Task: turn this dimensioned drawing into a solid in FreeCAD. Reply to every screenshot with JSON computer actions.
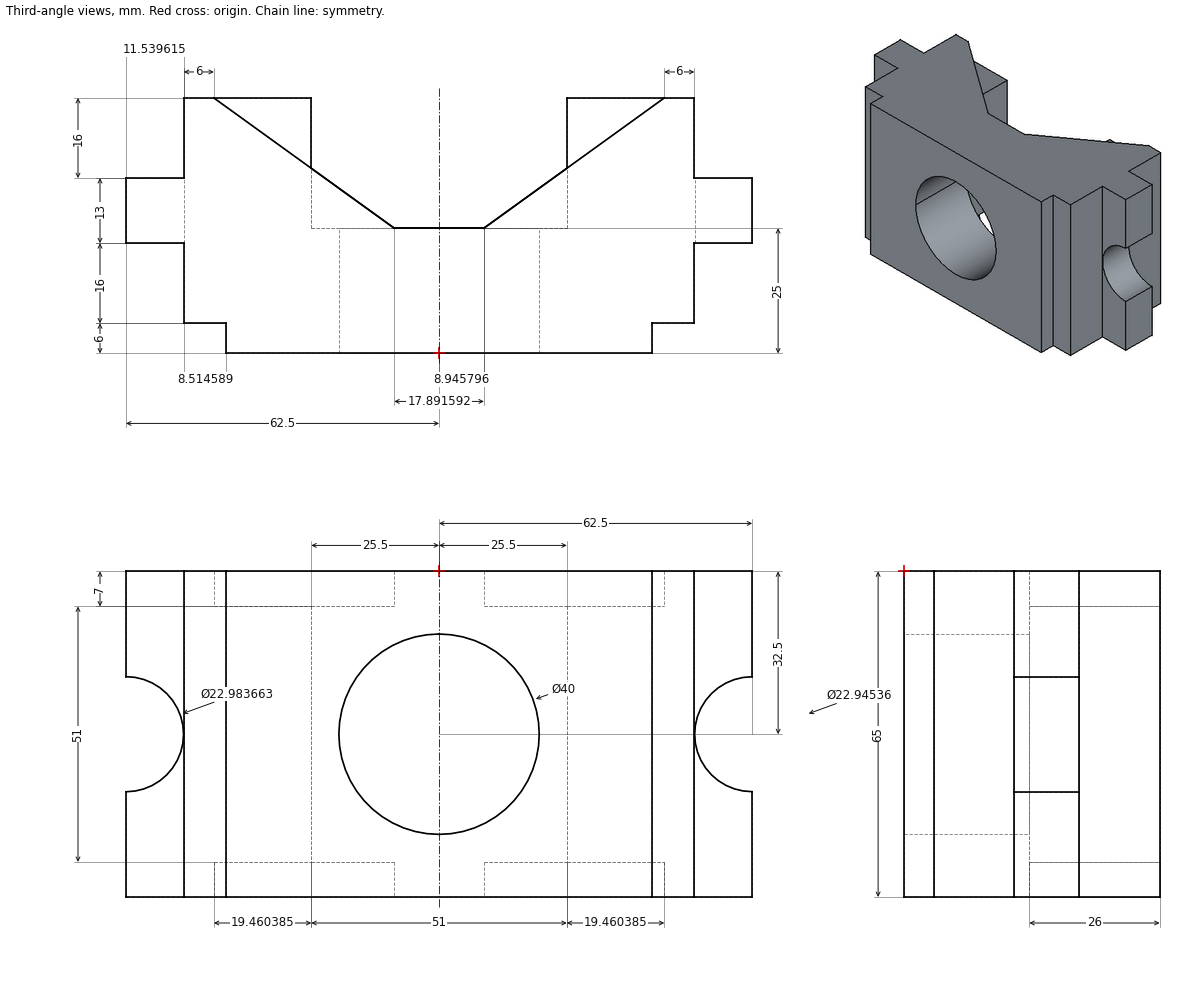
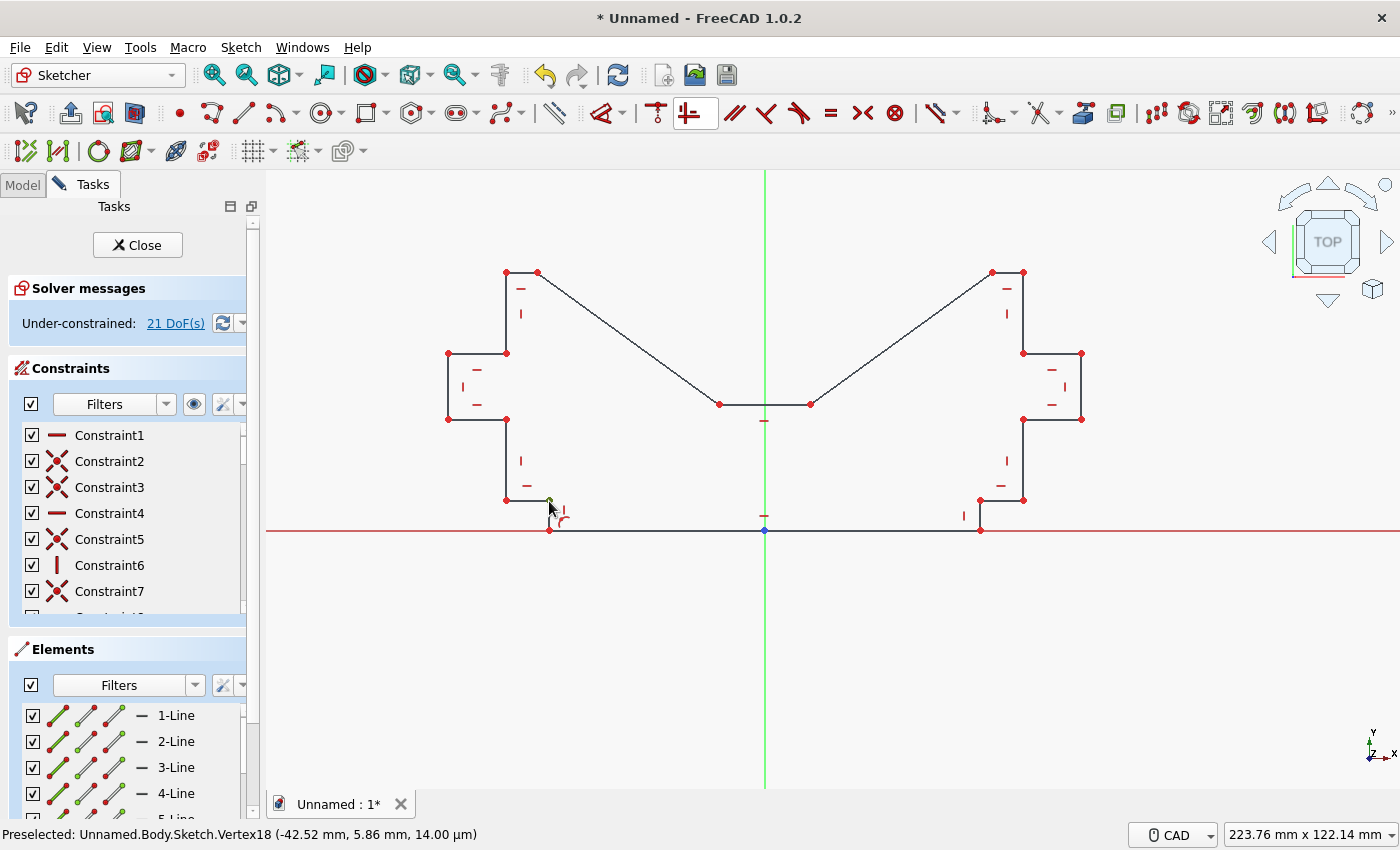
{"action": "left_click", "coordinate": [980, 501]}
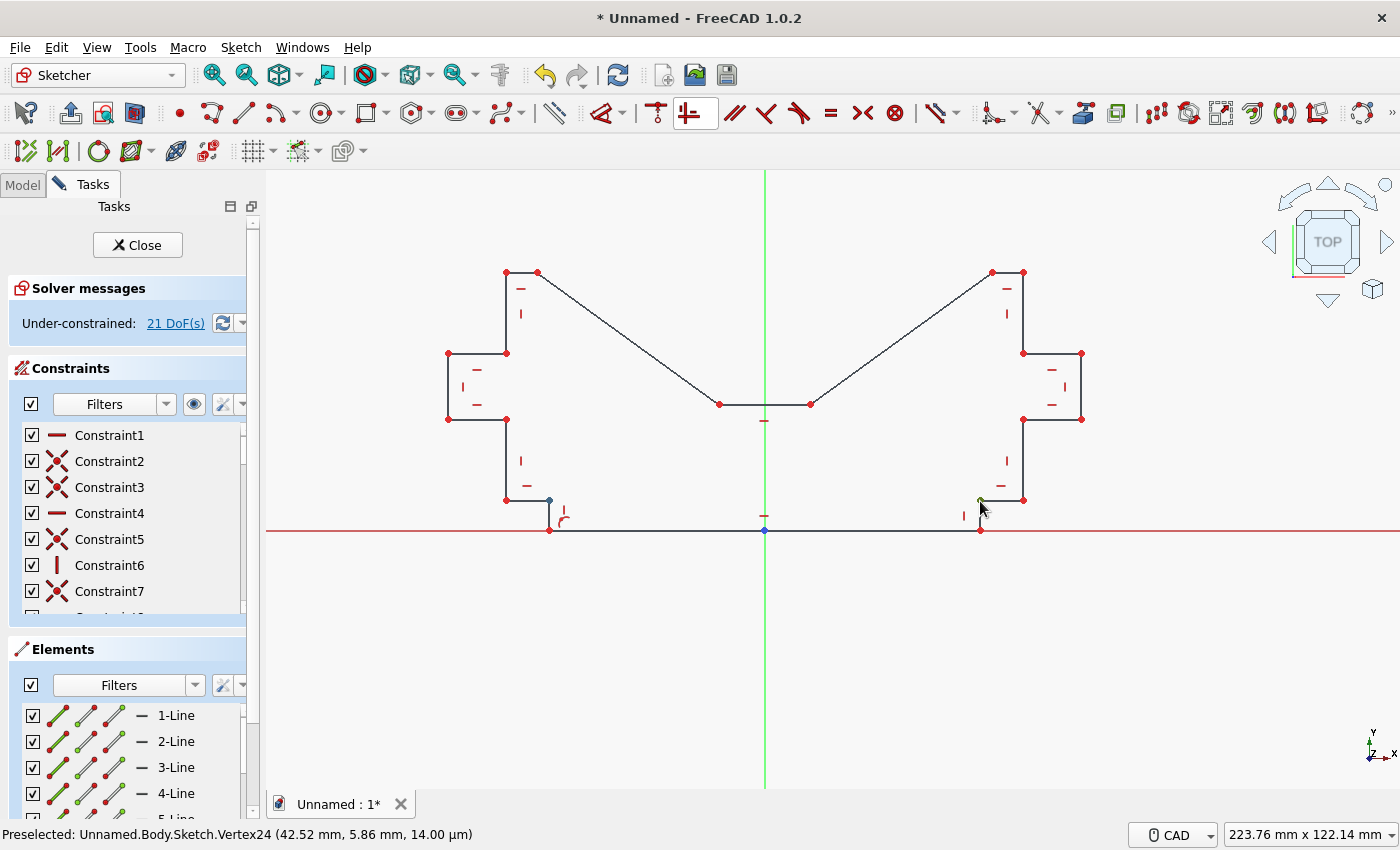
{"action": "left_click", "coordinate": [765, 721]}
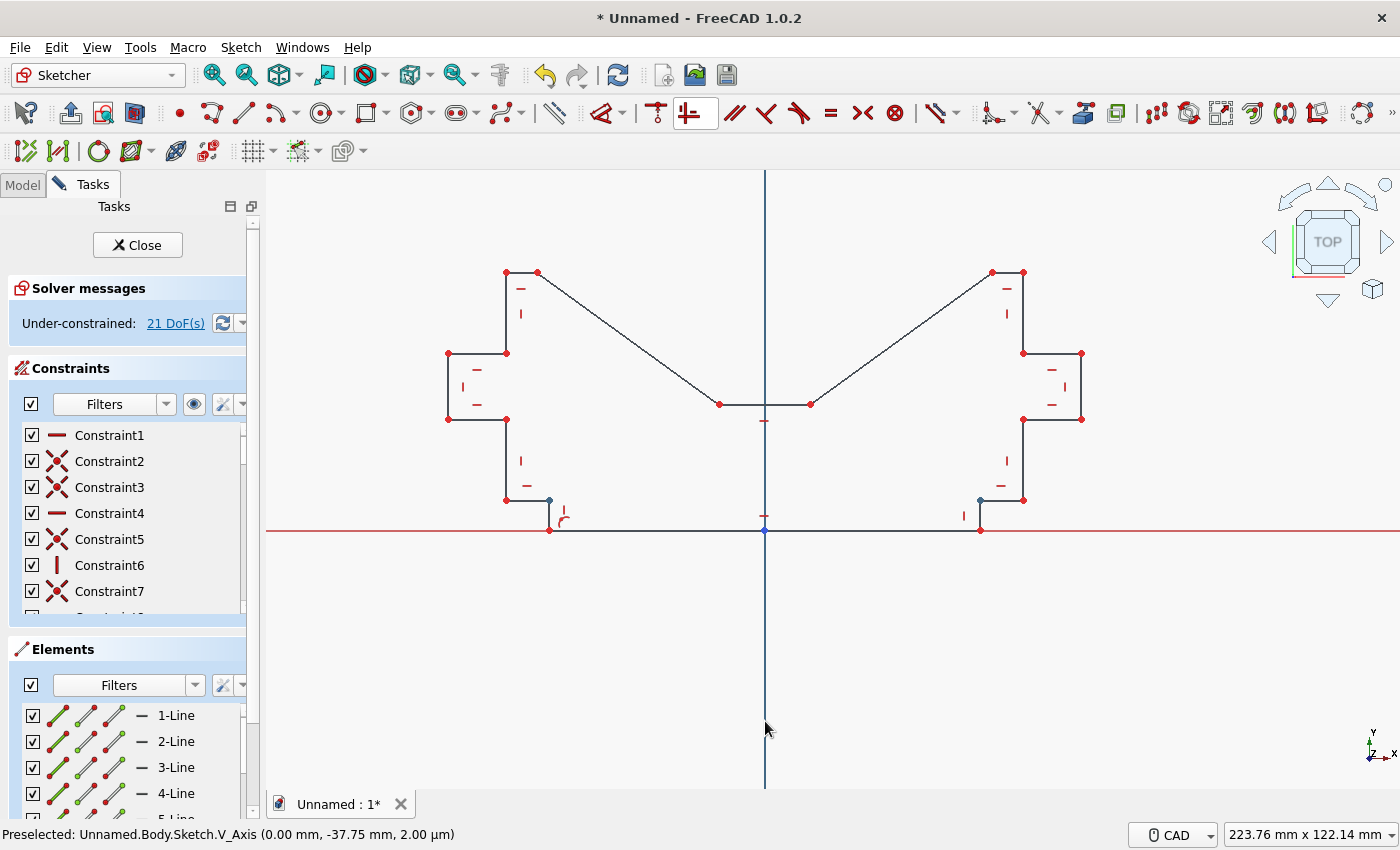
{"action": "left_click", "coordinate": [864, 114]}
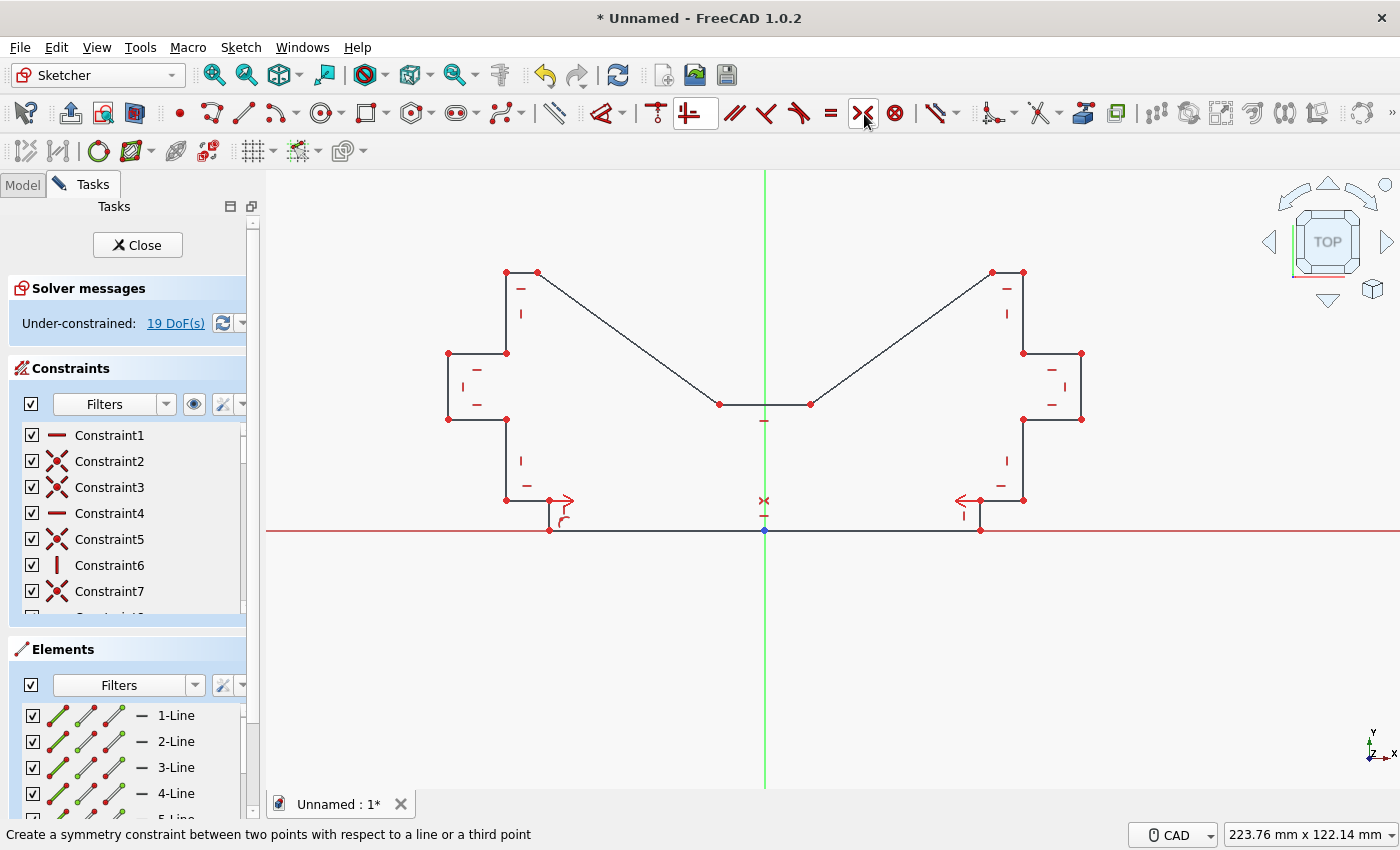
{"action": "left_click", "coordinate": [506, 420]}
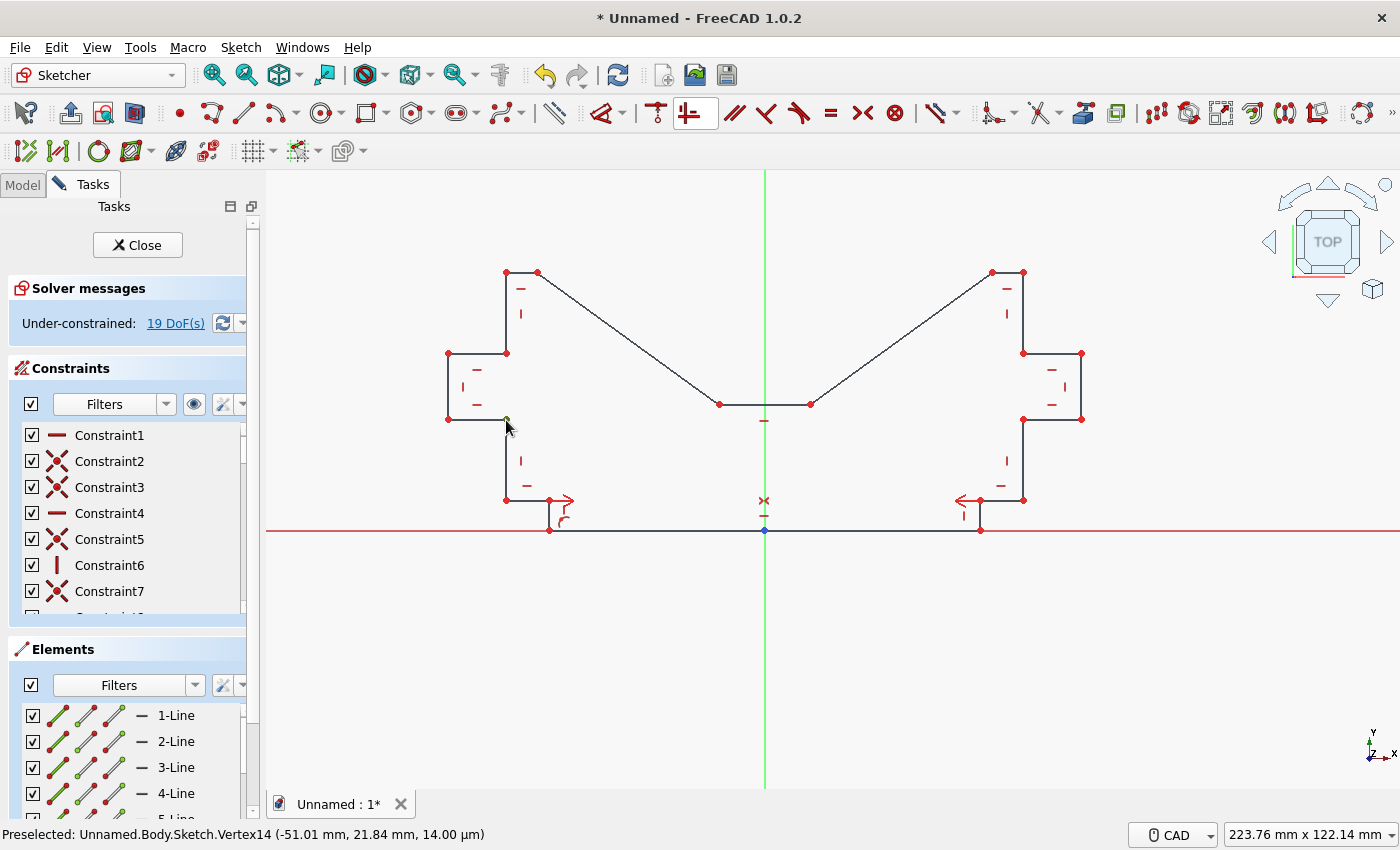
{"action": "left_click", "coordinate": [1023, 420]}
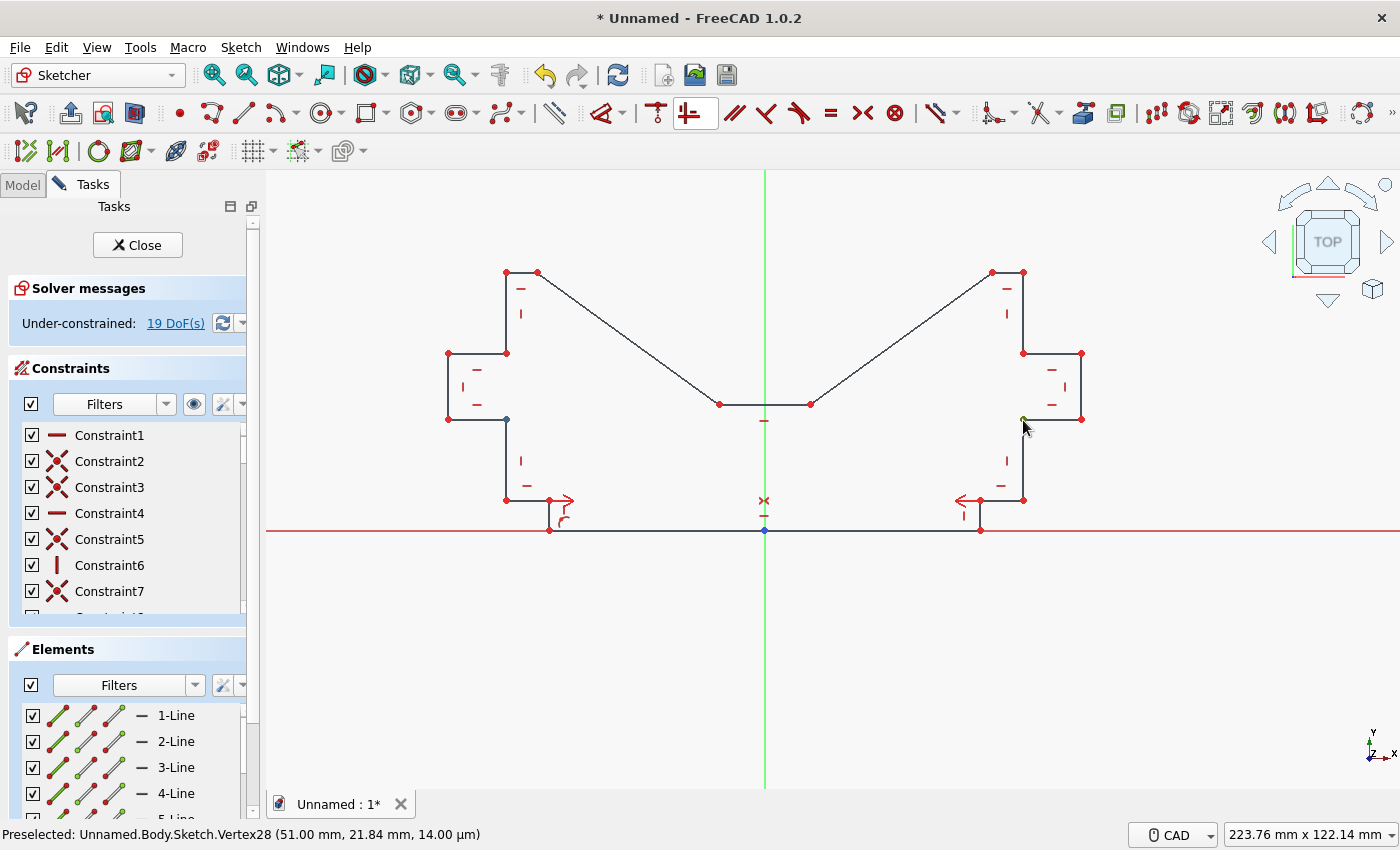
{"action": "left_click", "coordinate": [765, 721]}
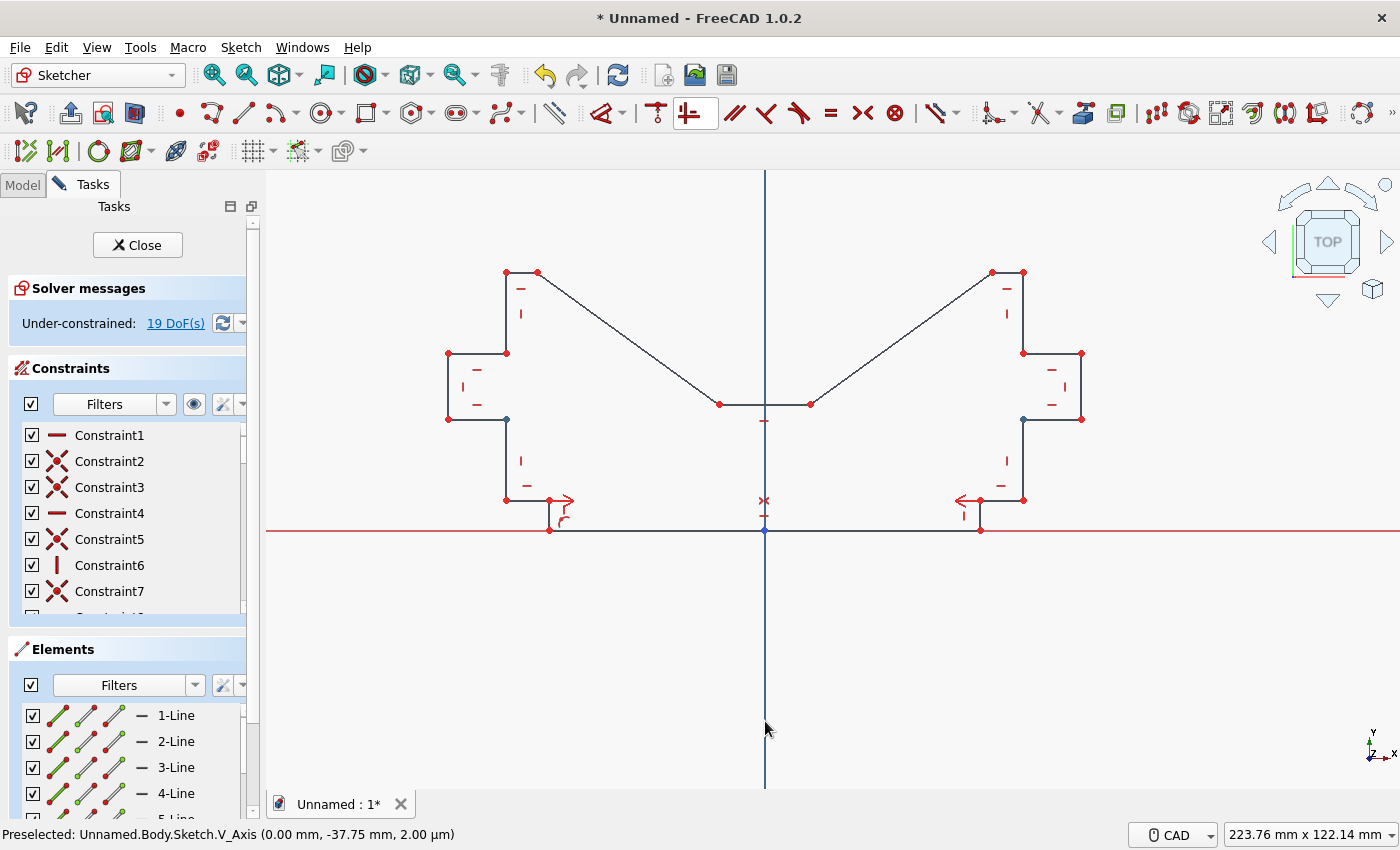
{"action": "left_click", "coordinate": [864, 114]}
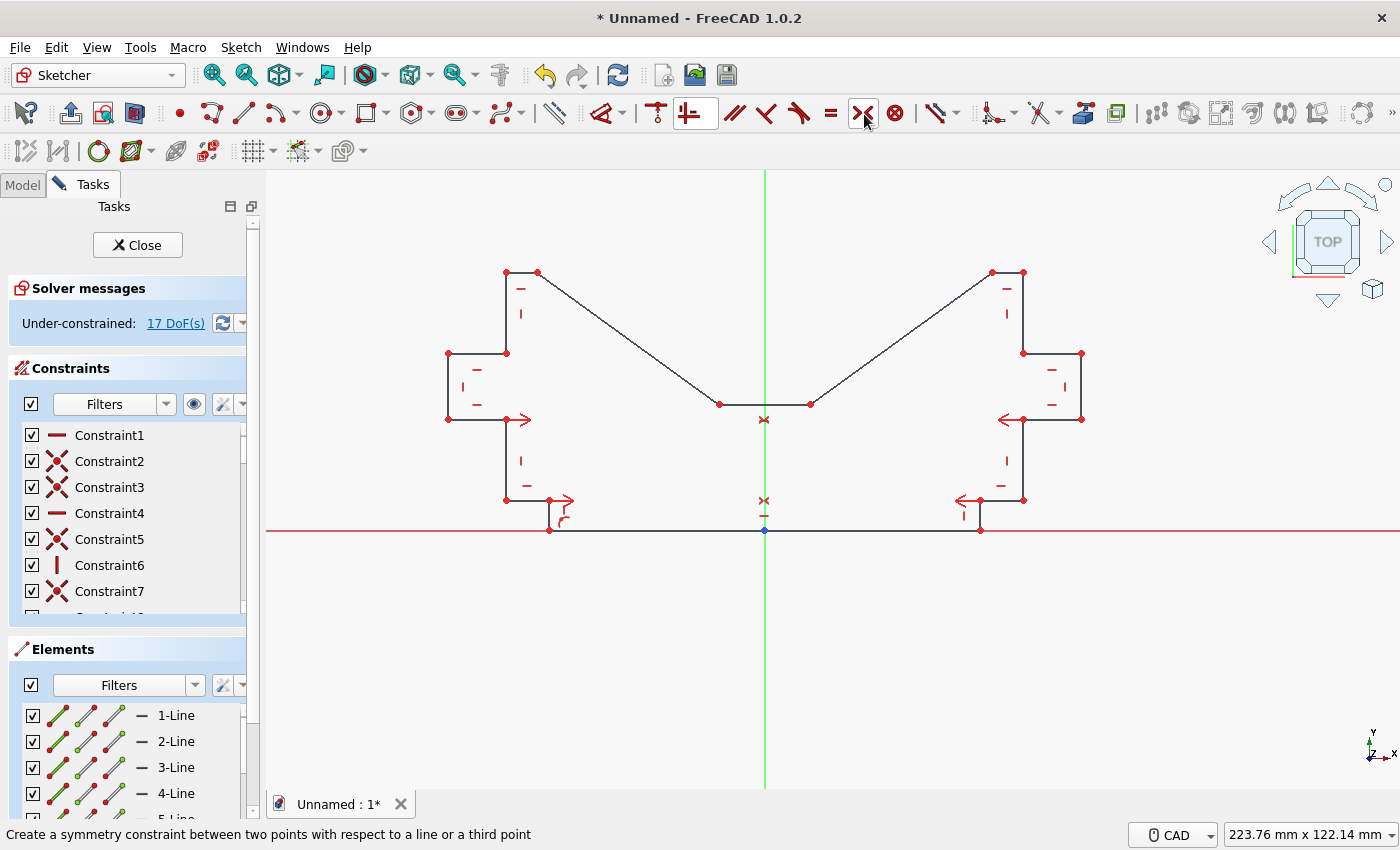
{"action": "left_click", "coordinate": [448, 354]}